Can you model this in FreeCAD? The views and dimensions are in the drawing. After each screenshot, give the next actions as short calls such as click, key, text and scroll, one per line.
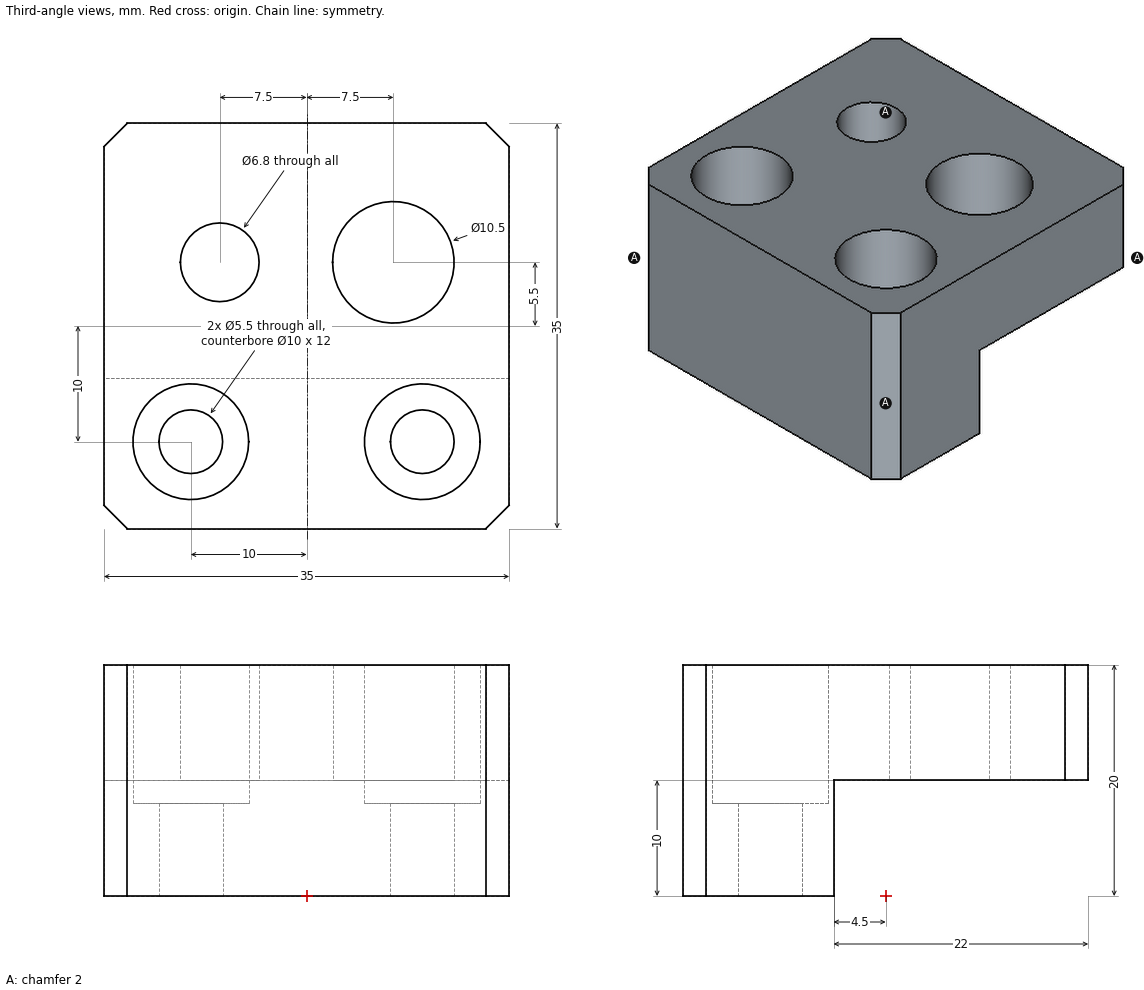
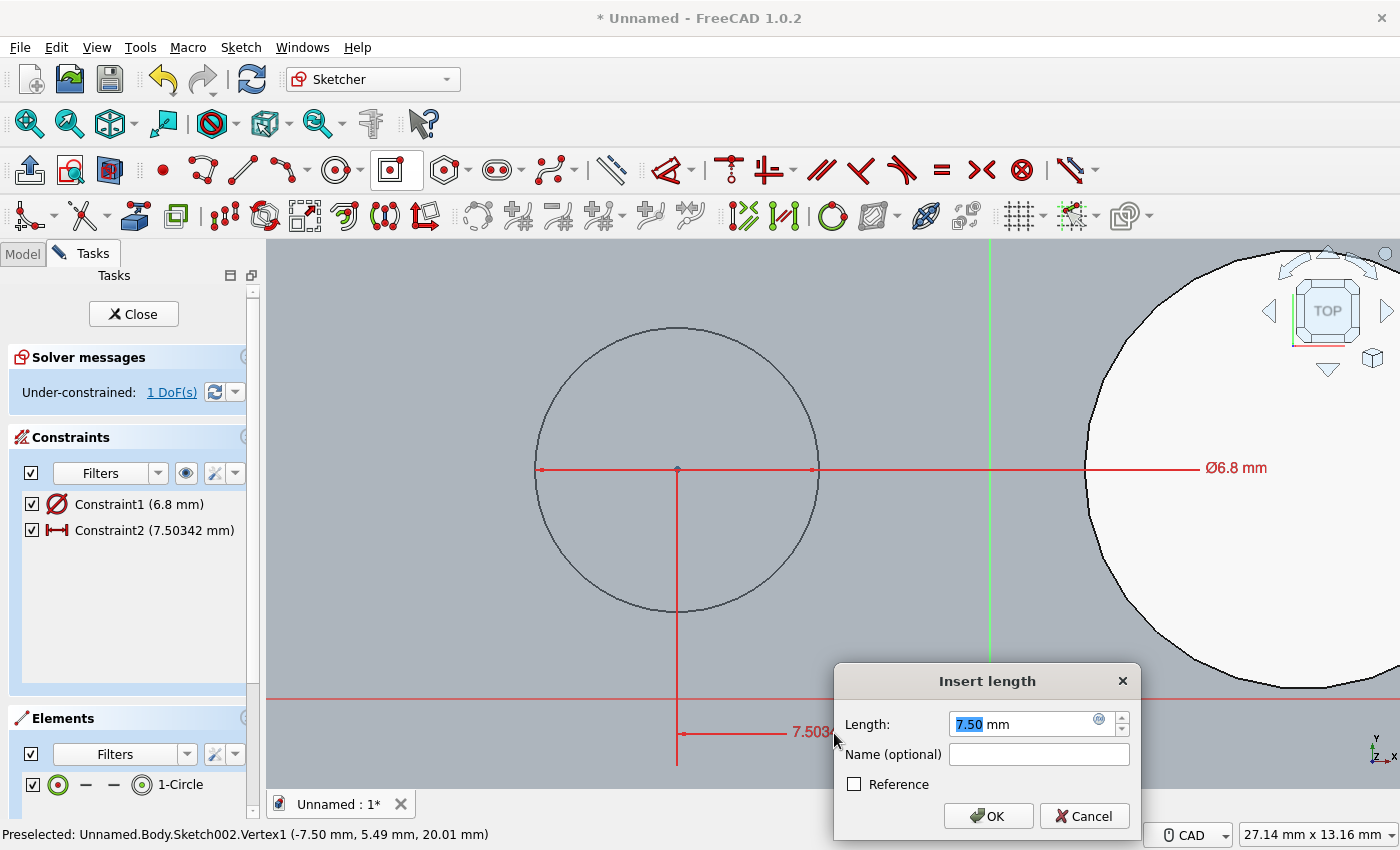
text(7.5)
key(Return)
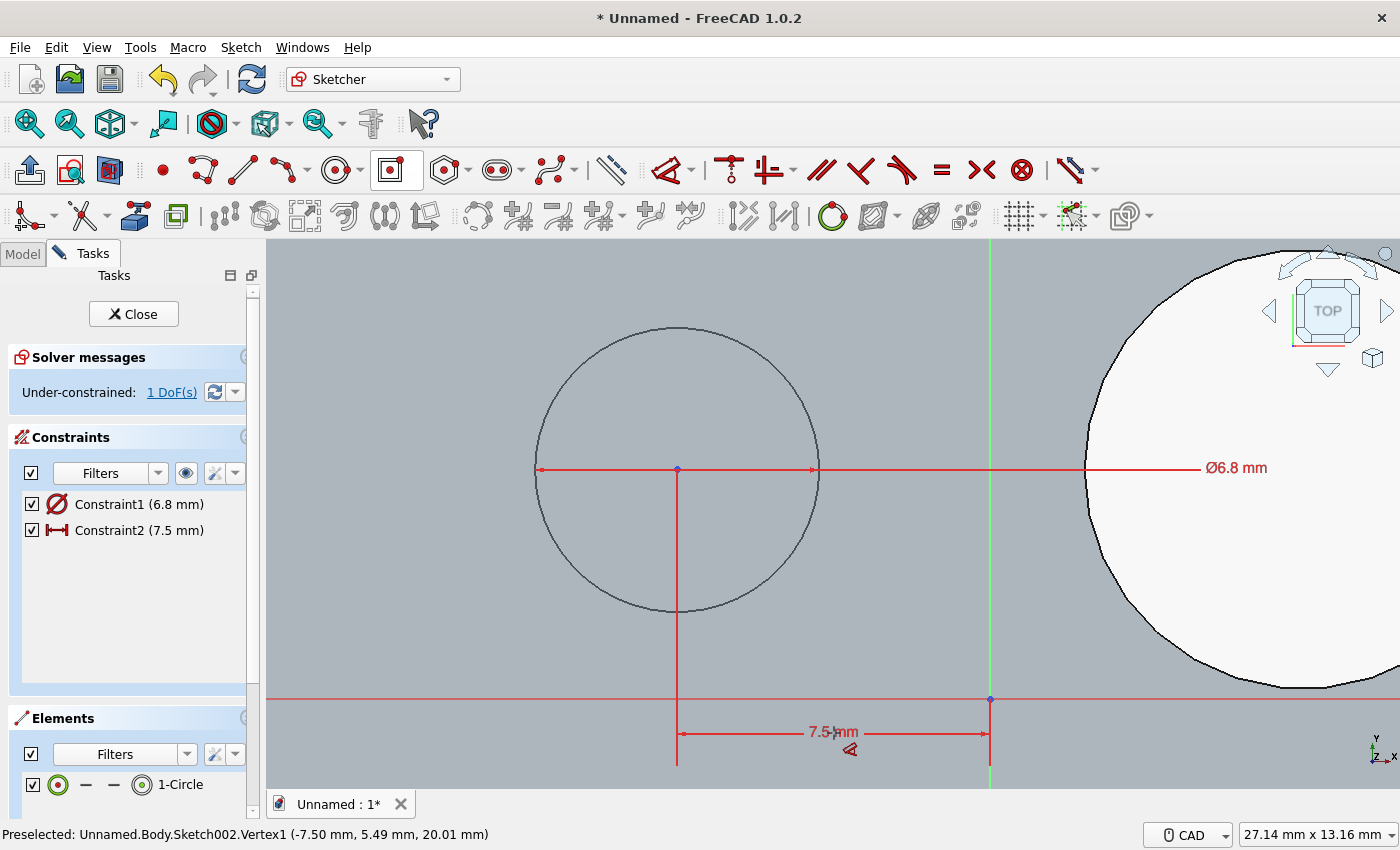
click(677, 470)
click(1024, 585)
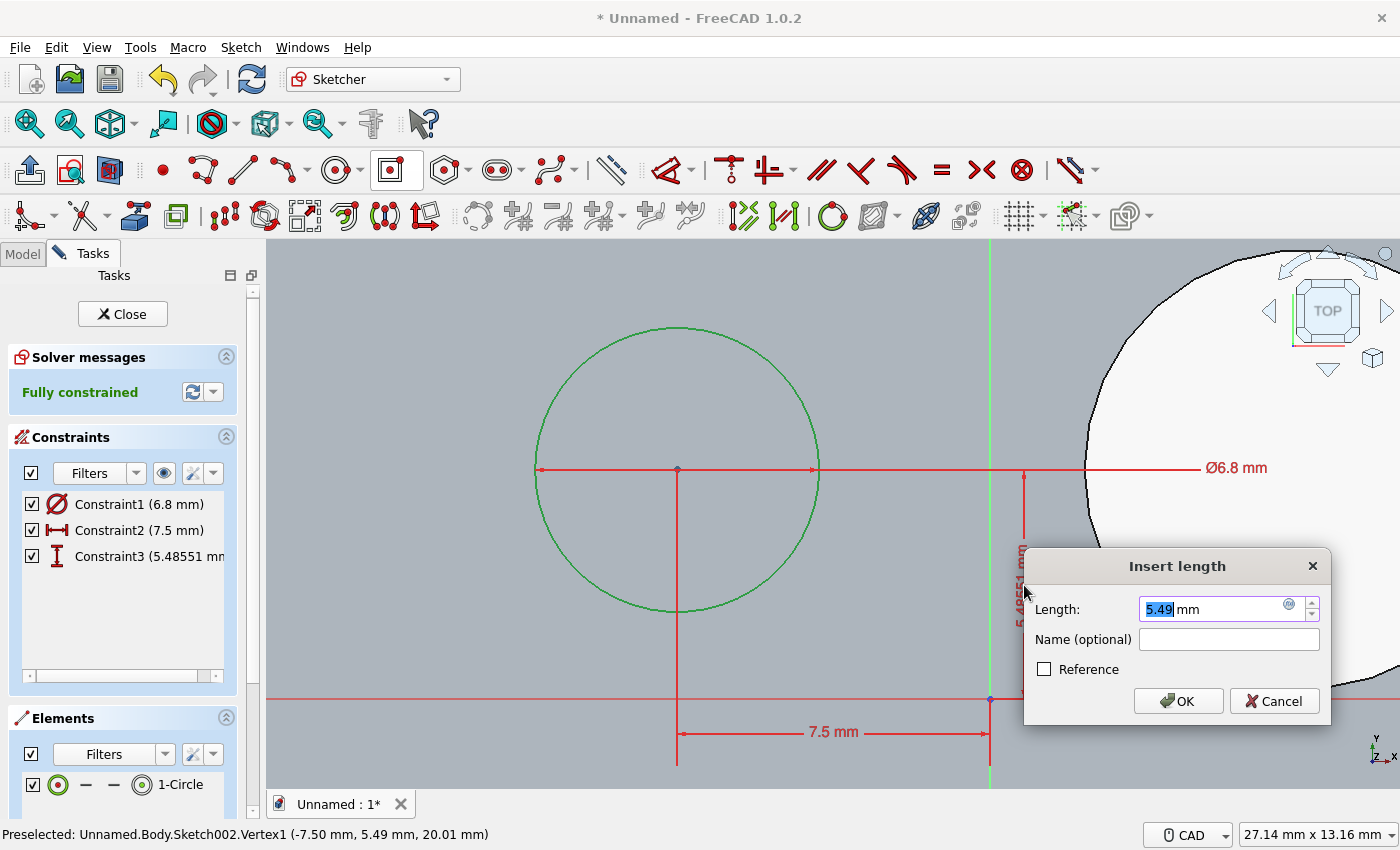
text(5.5)
key(Return)
key(Escape)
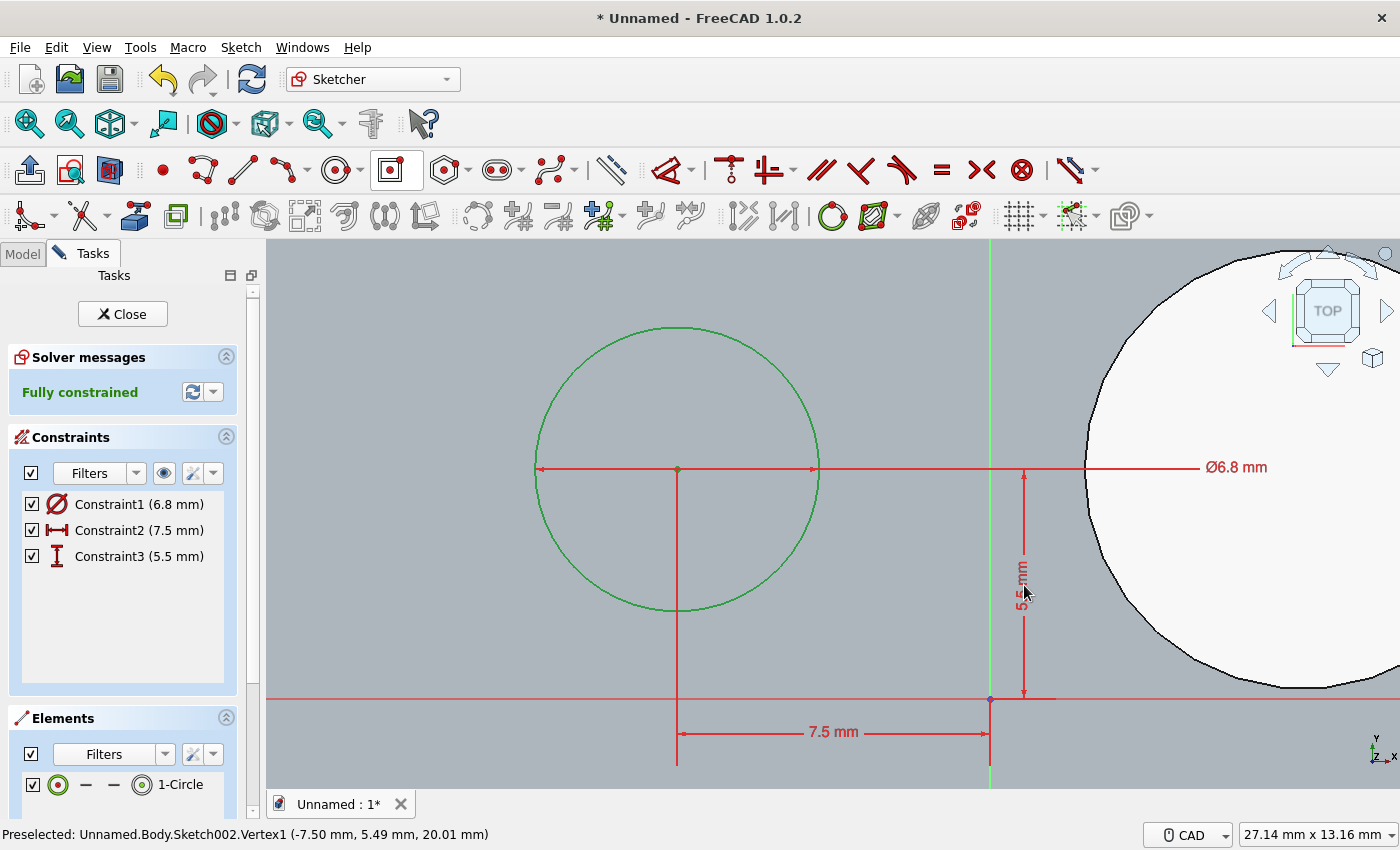
click(123, 314)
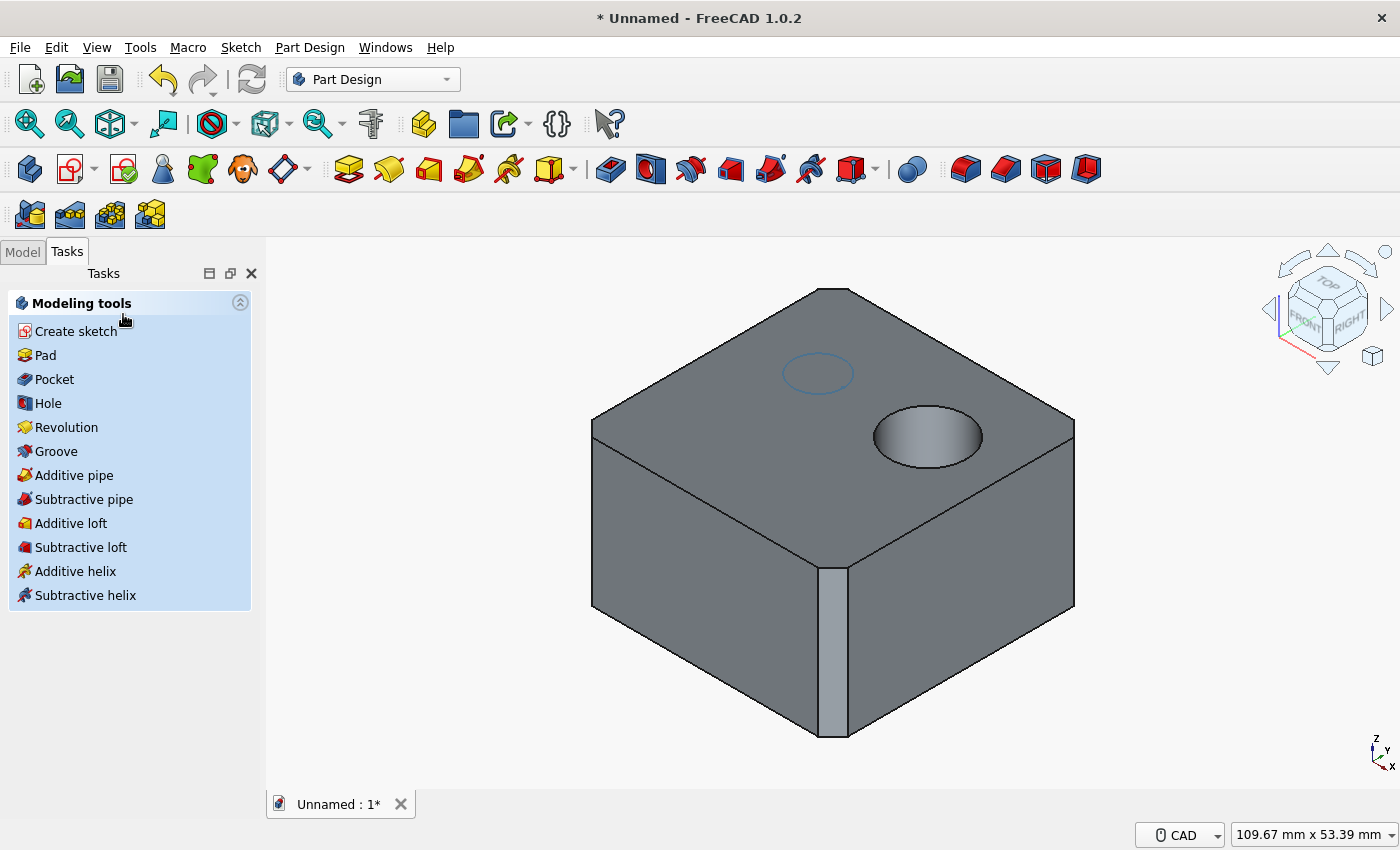
click(652, 170)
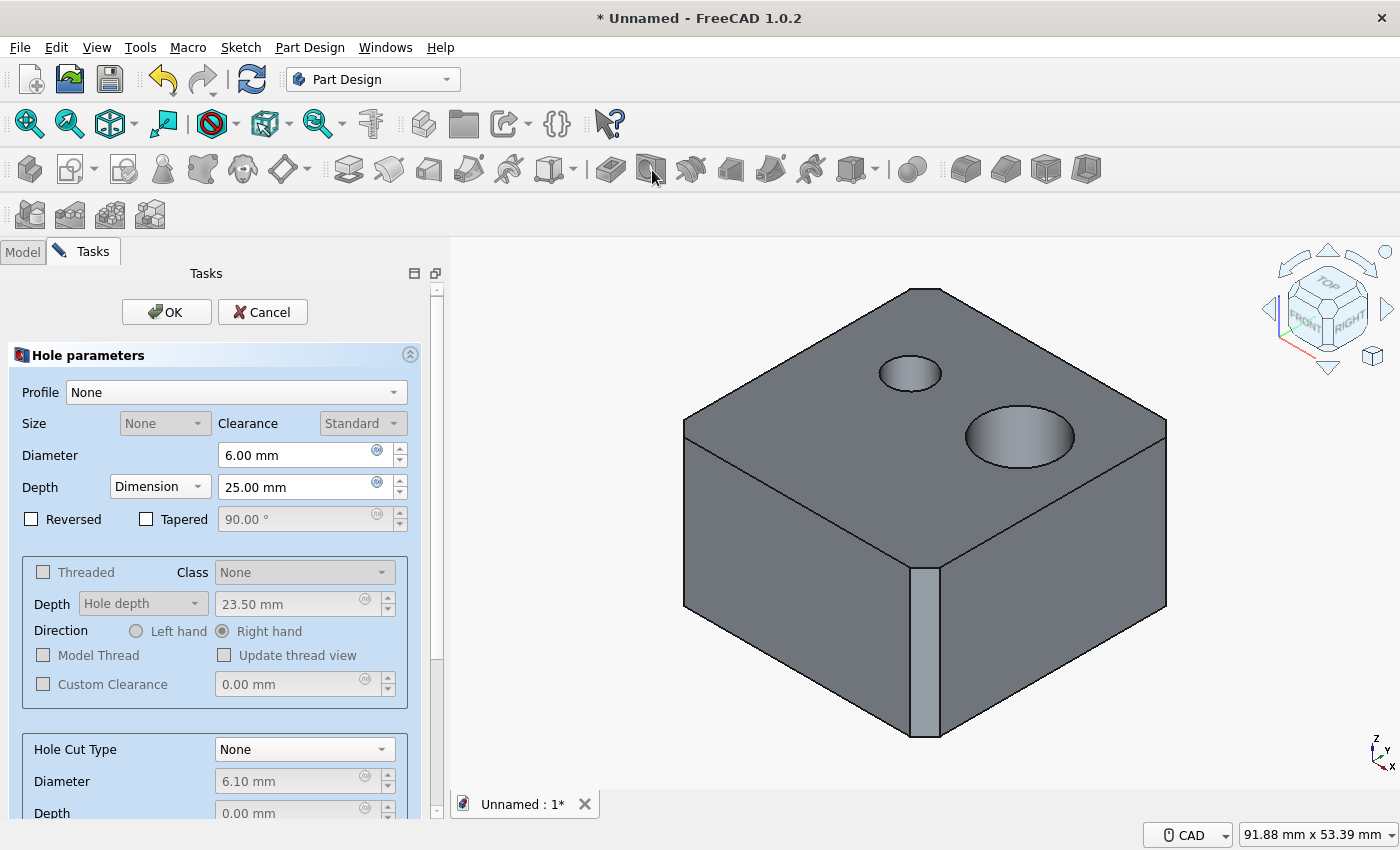
triple_click(305, 455)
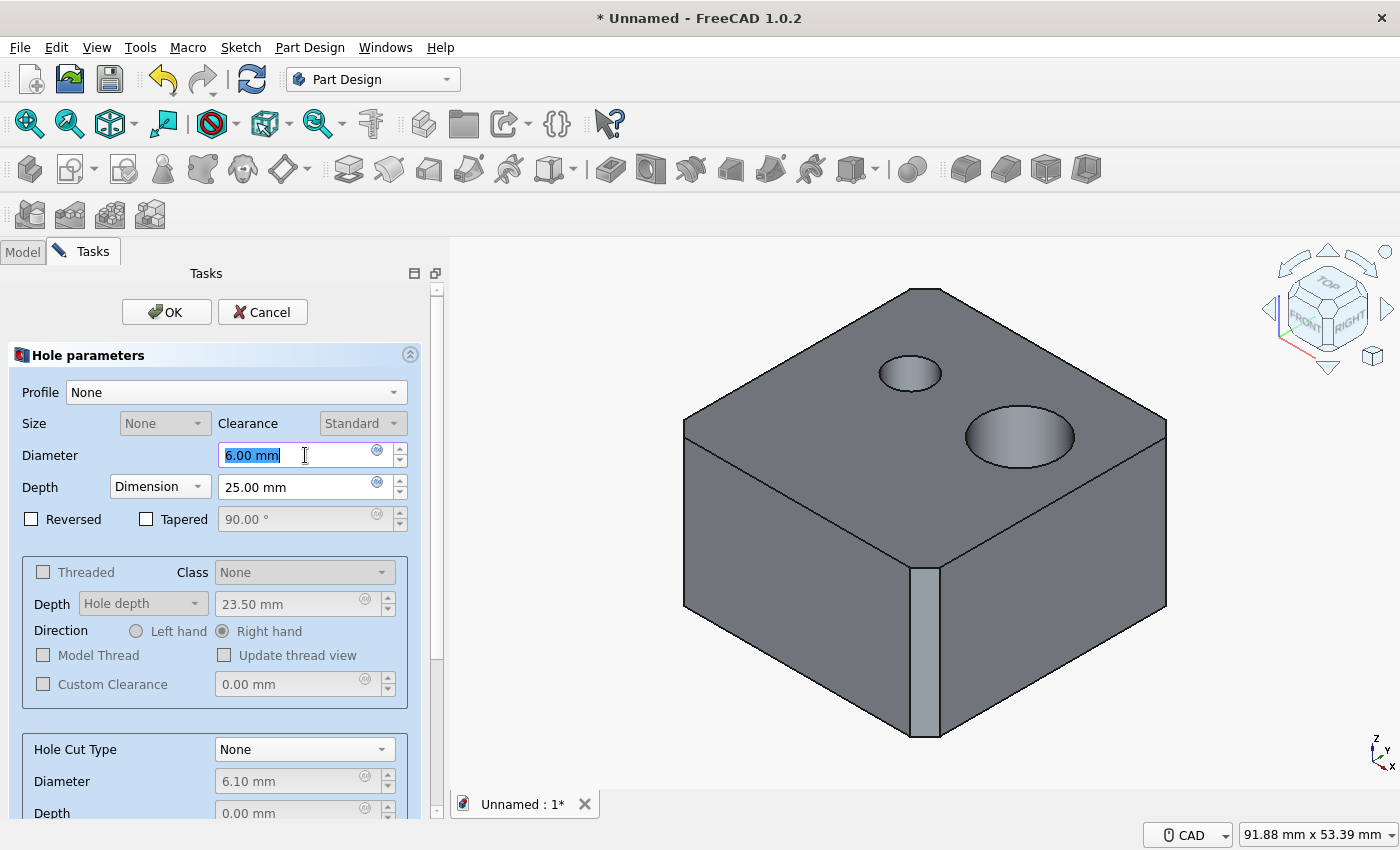
text(6.8)
key(Tab)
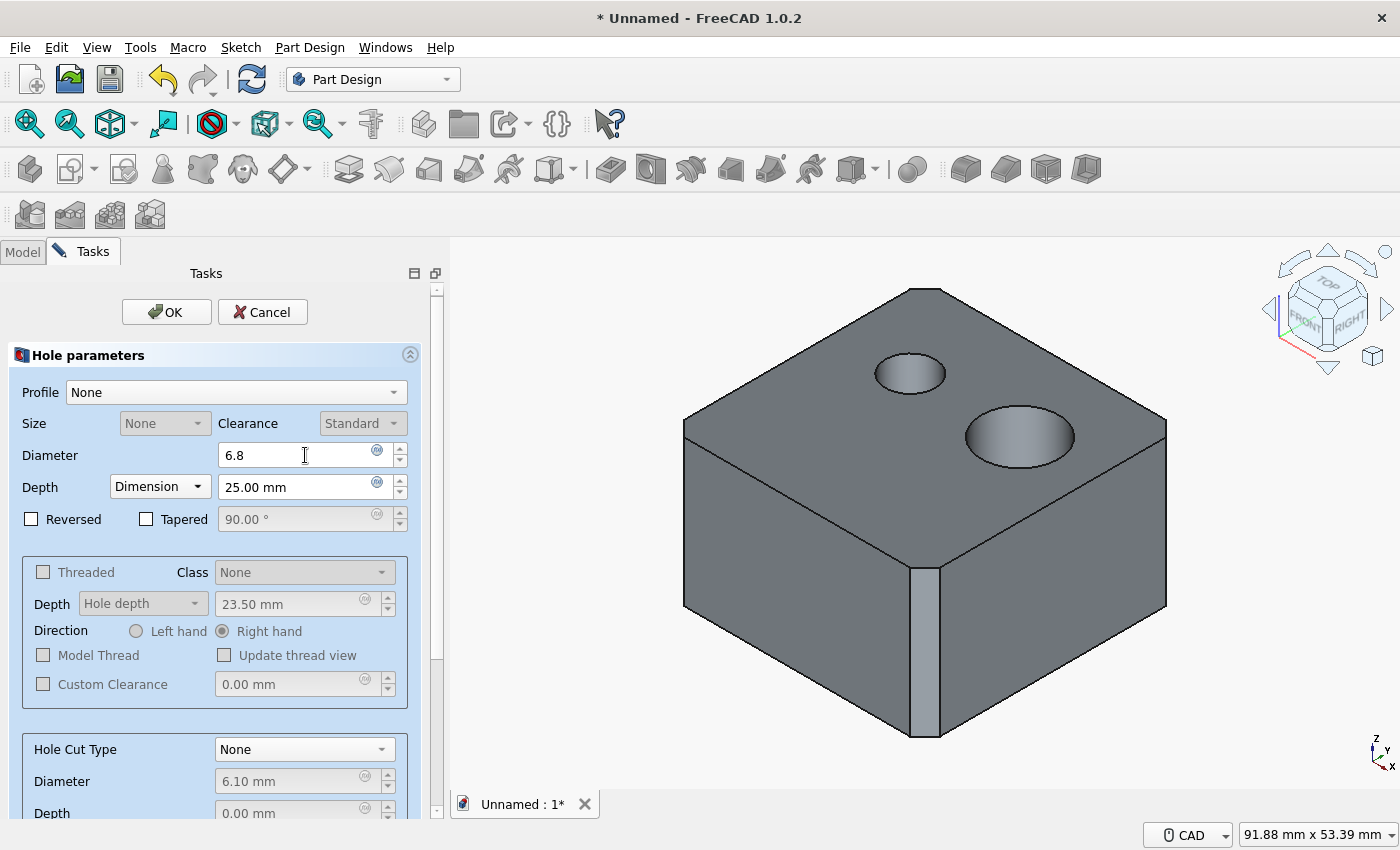
click(161, 486)